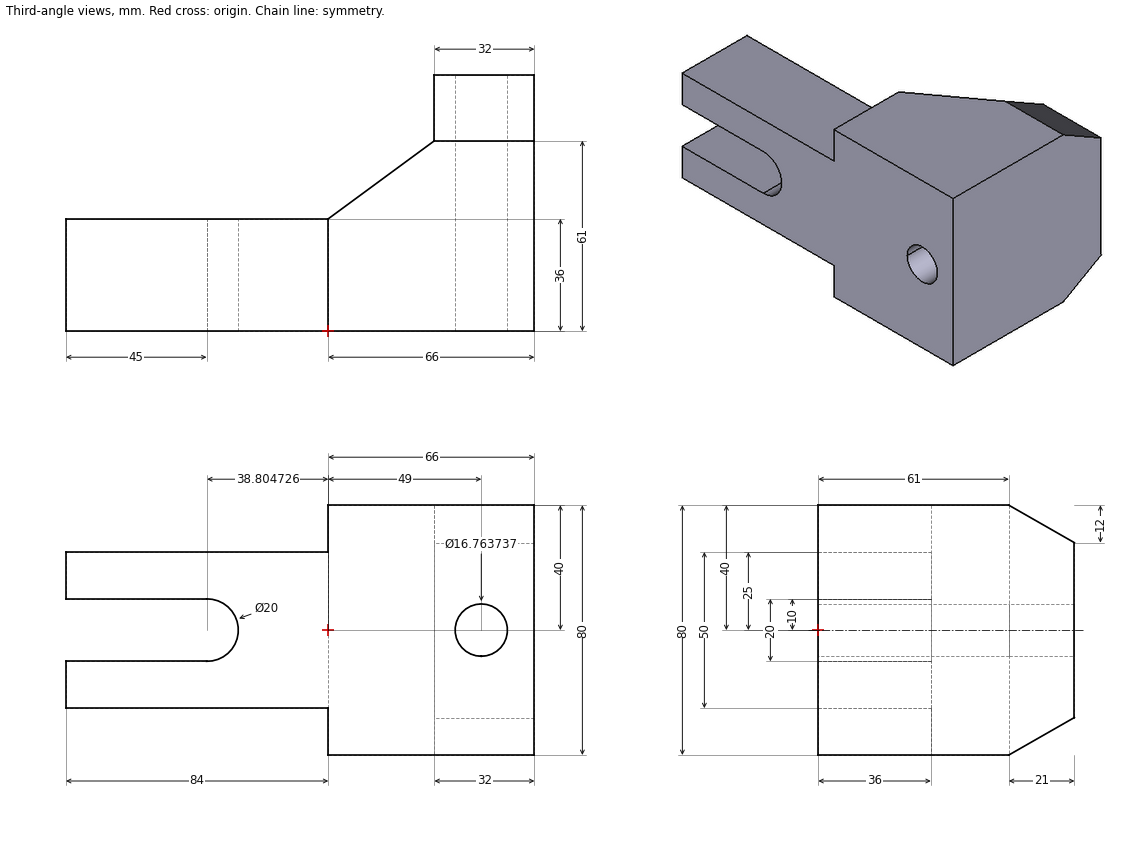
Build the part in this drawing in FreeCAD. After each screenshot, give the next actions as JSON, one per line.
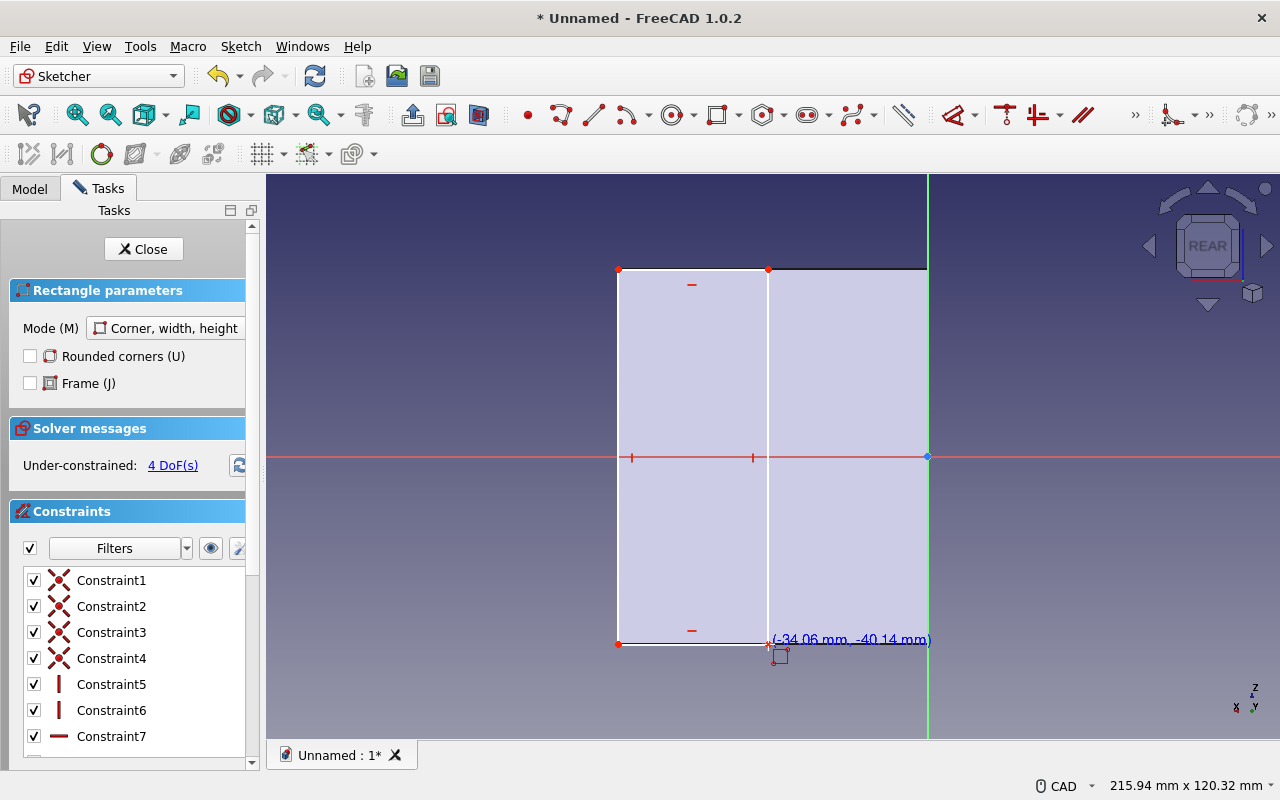
{"action": "key", "text": "g c"}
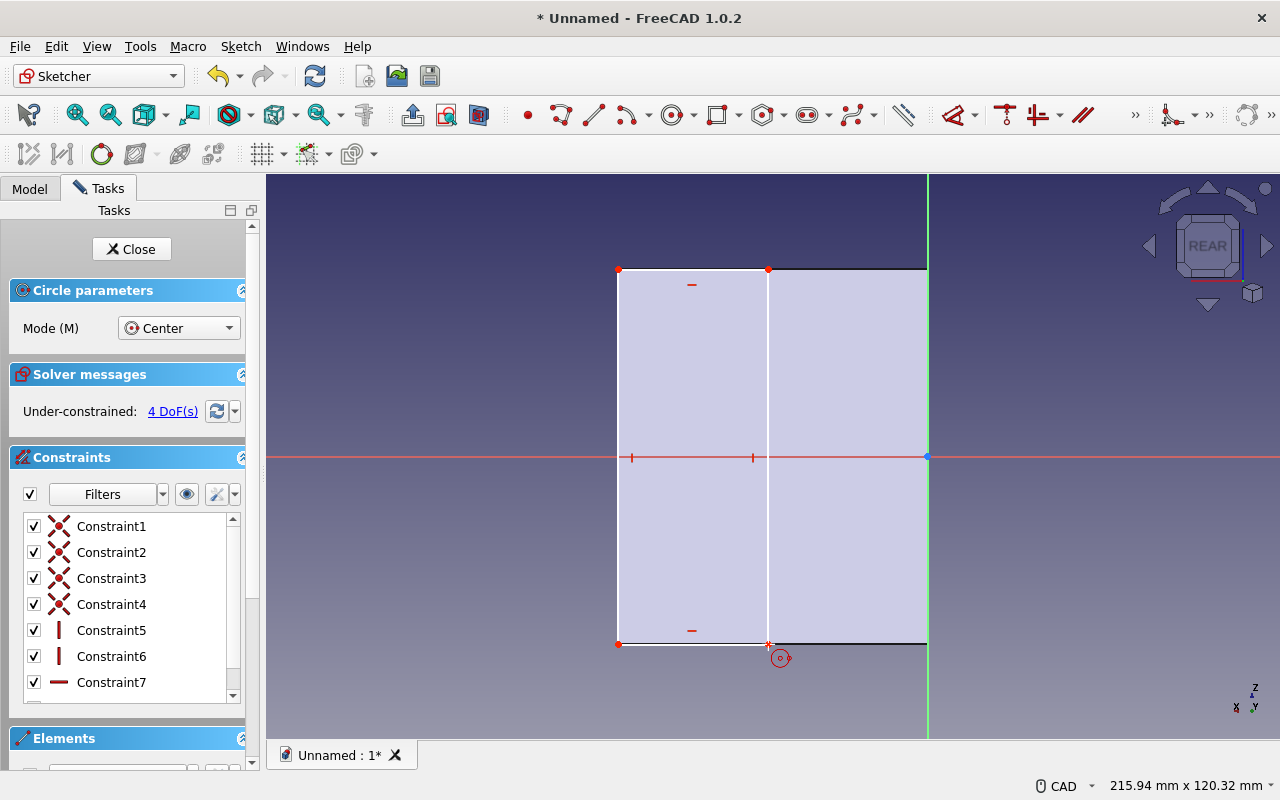
{"action": "left_click", "coordinate": [698, 457]}
{"action": "left_click", "coordinate": [726, 429]}
{"action": "key", "text": "Escape"}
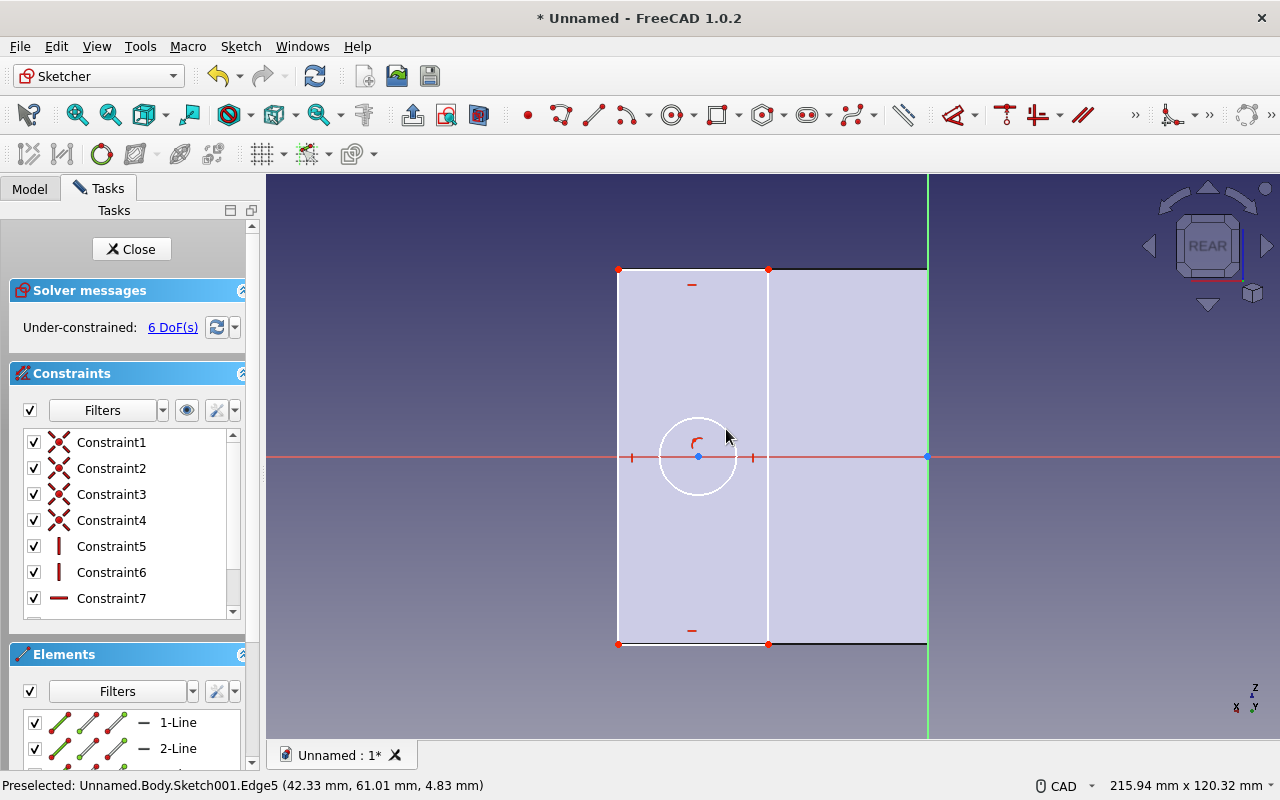
{"action": "key", "text": "d"}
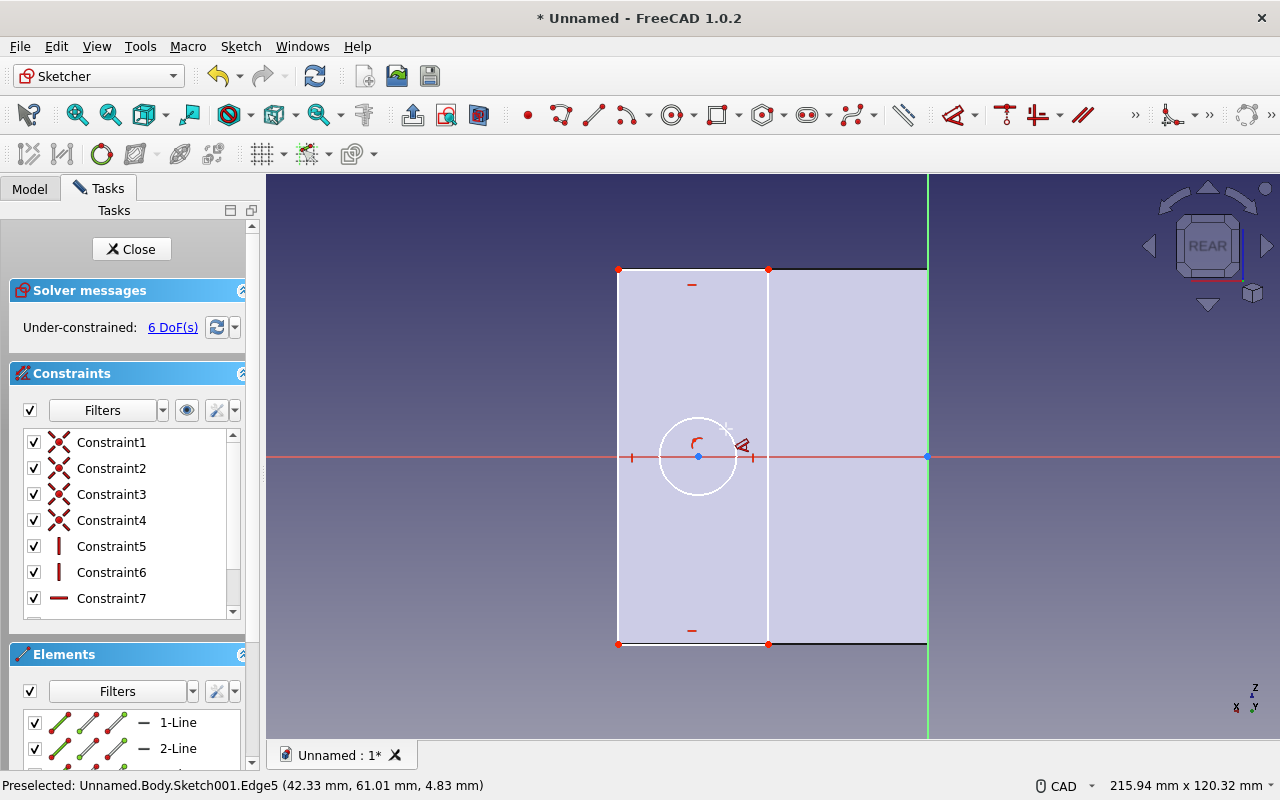
{"action": "left_click", "coordinate": [725, 429]}
{"action": "left_click", "coordinate": [747, 406]}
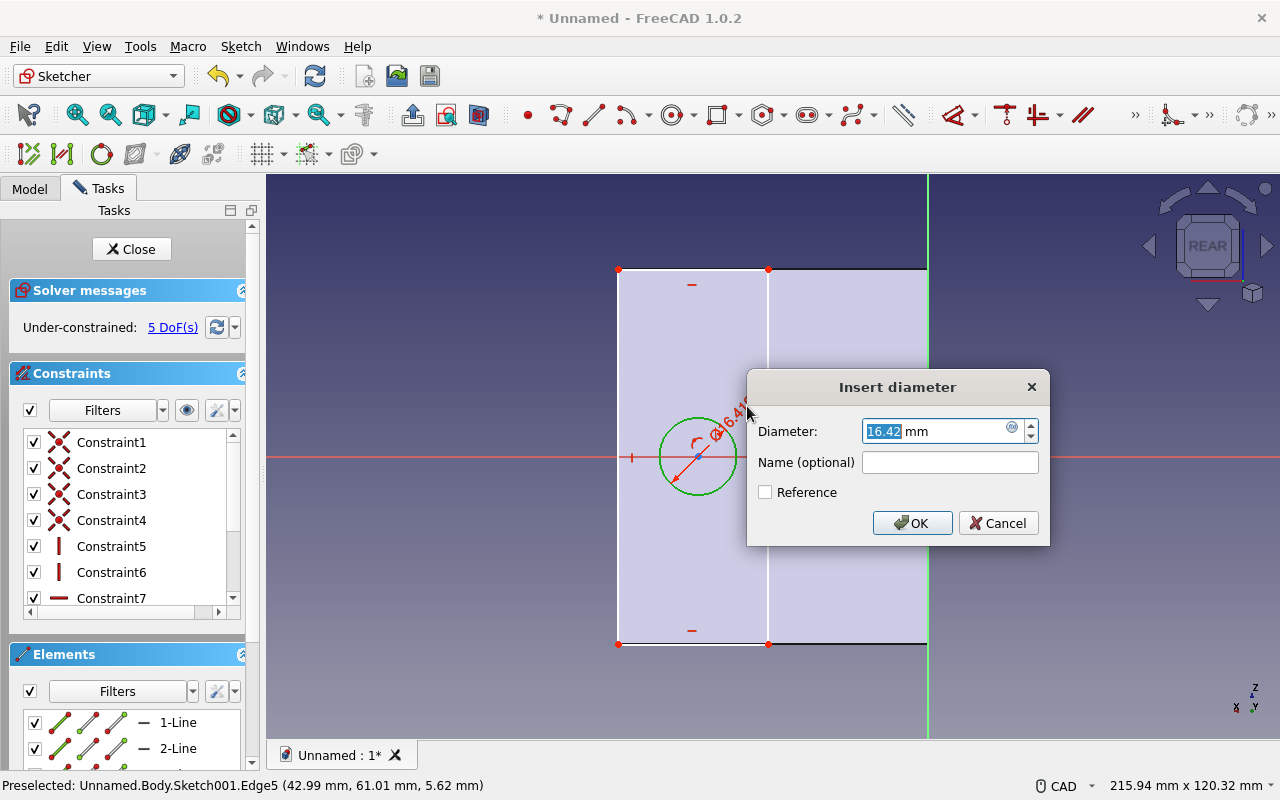
{"action": "type", "text": "16.763737"}
{"action": "key", "text": "Return"}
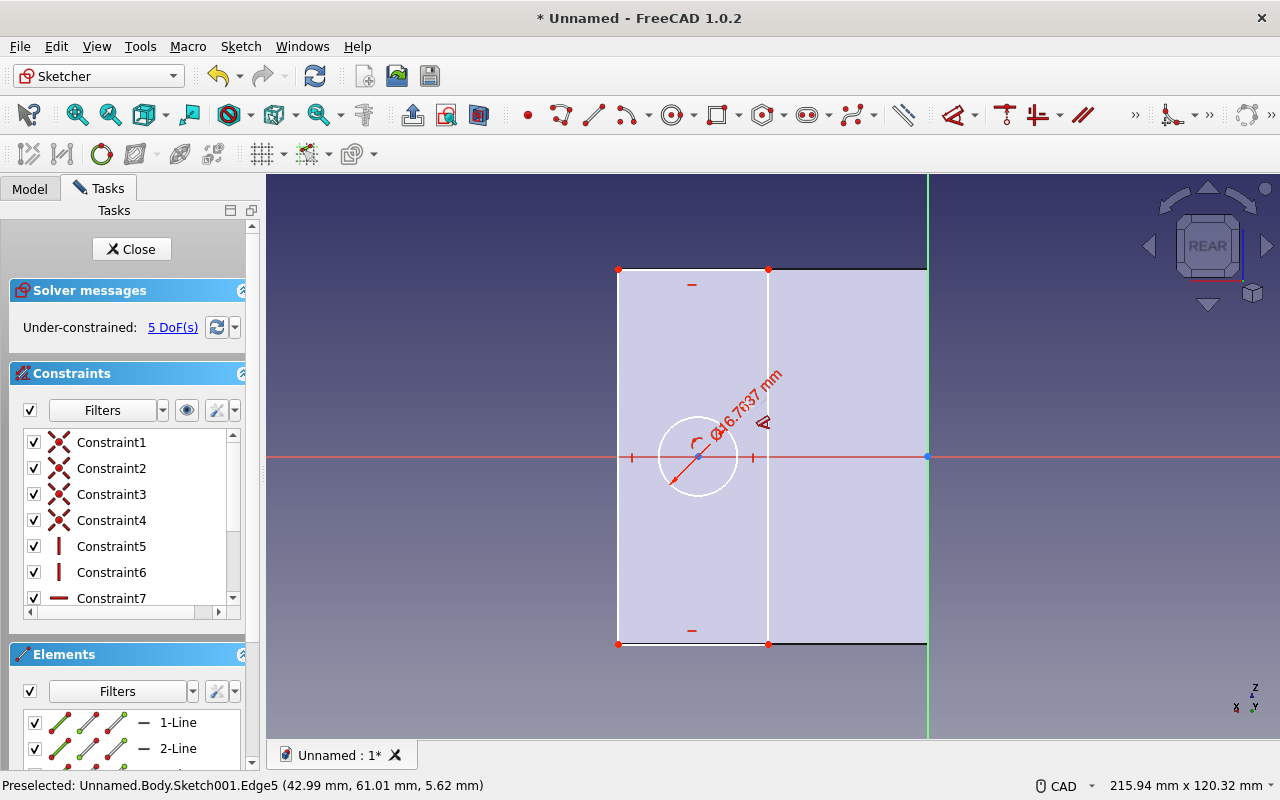
{"action": "left_click", "coordinate": [618, 382]}
{"action": "left_click", "coordinate": [584, 371]}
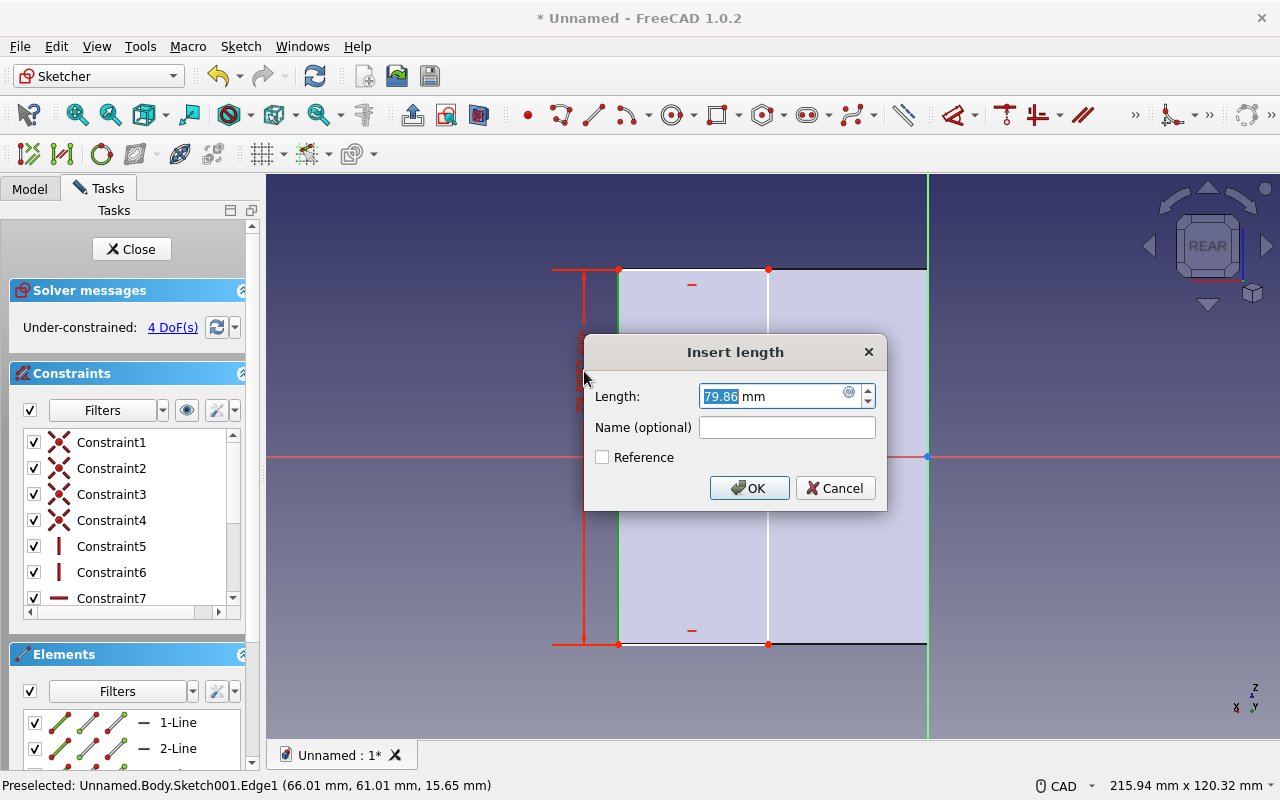
{"action": "type", "text": "80"}
{"action": "key", "text": "Return"}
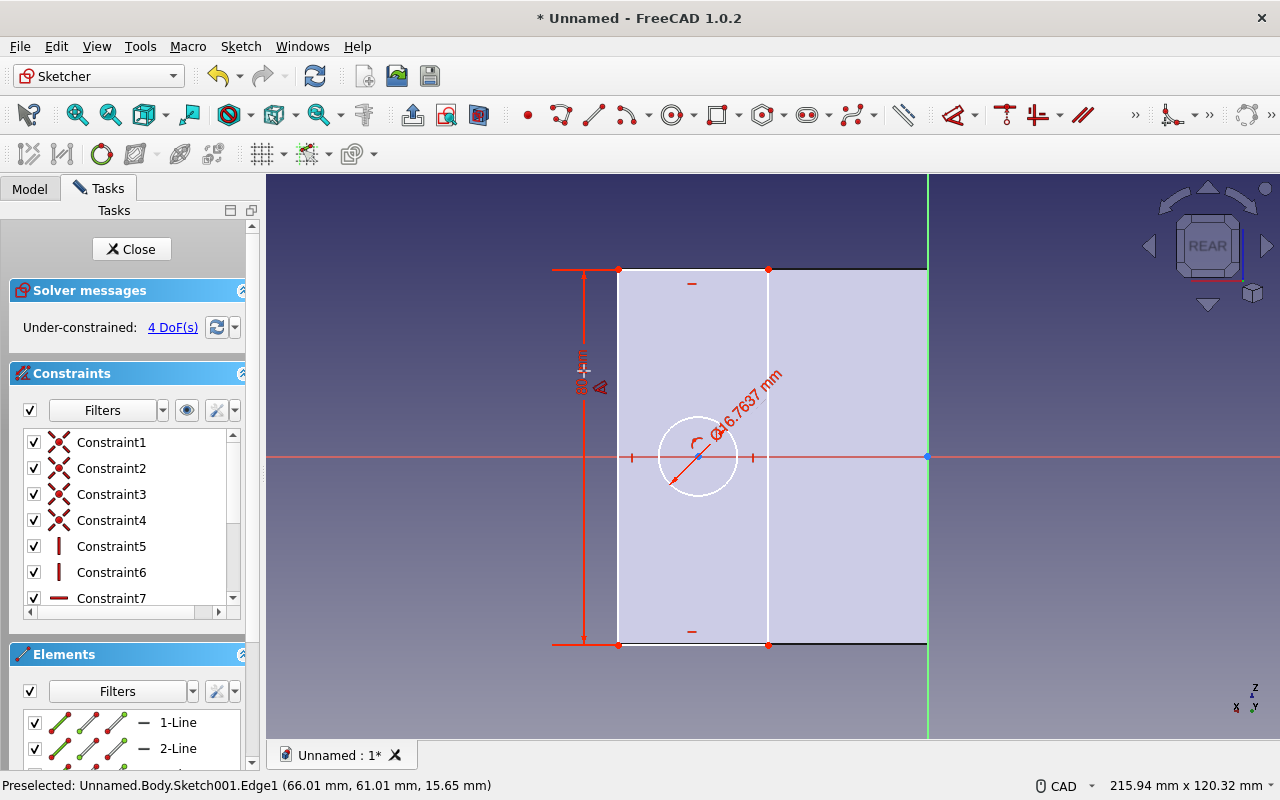
{"action": "left_click", "coordinate": [663, 645]}
{"action": "left_click", "coordinate": [693, 679]}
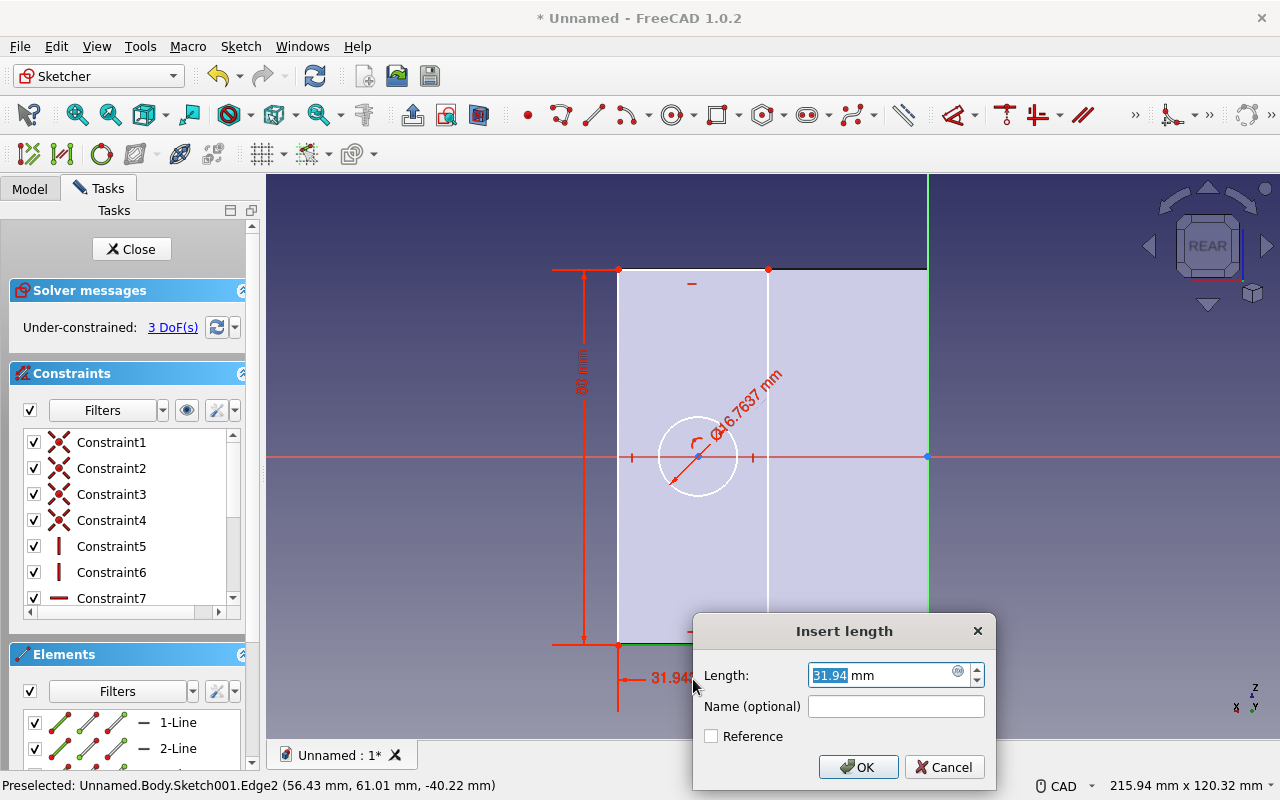
{"action": "type", "text": "32"}
{"action": "key", "text": "Return"}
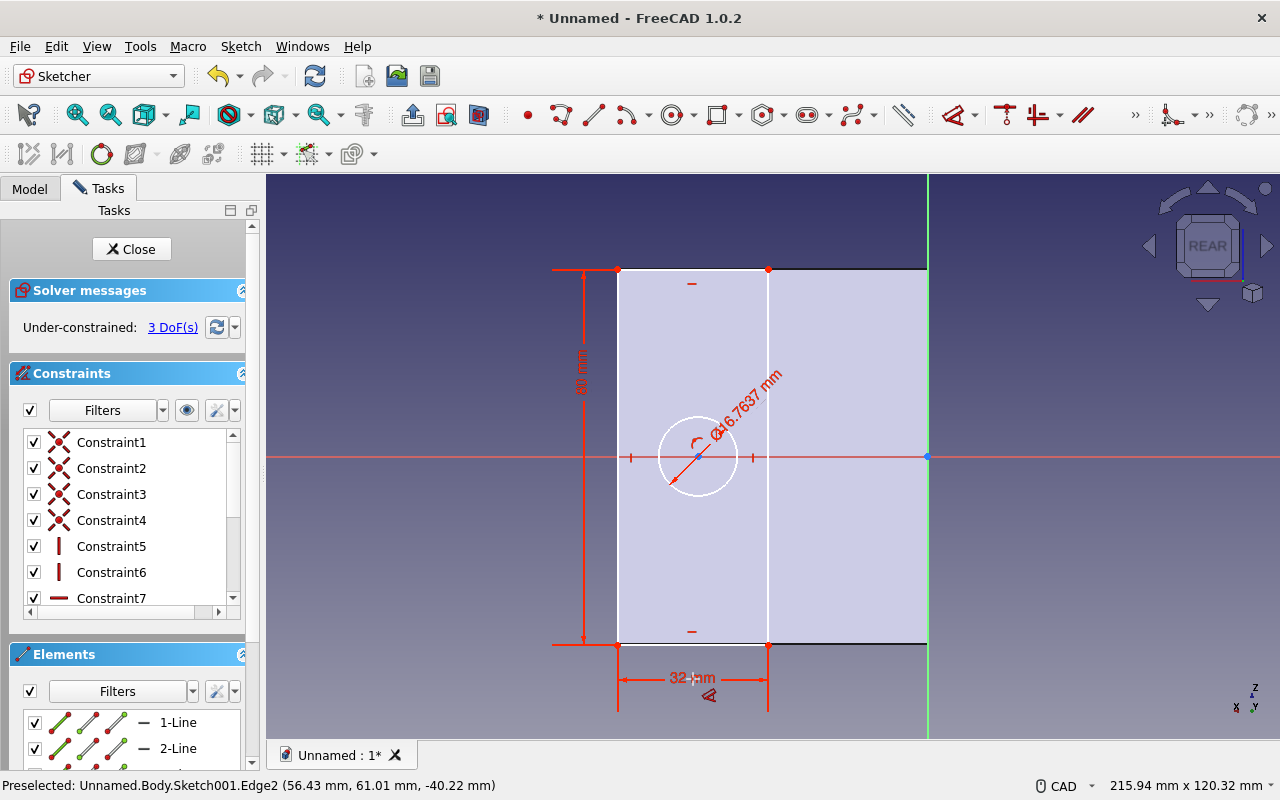
{"action": "left_click", "coordinate": [698, 457]}
{"action": "left_click", "coordinate": [813, 491]}